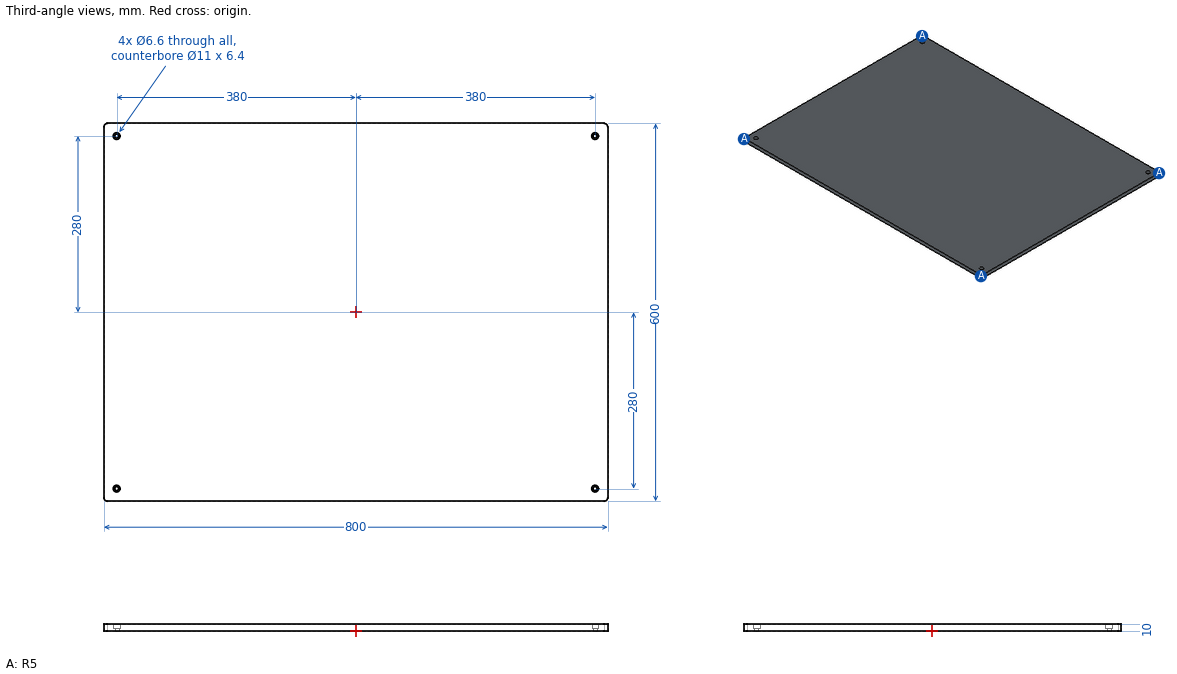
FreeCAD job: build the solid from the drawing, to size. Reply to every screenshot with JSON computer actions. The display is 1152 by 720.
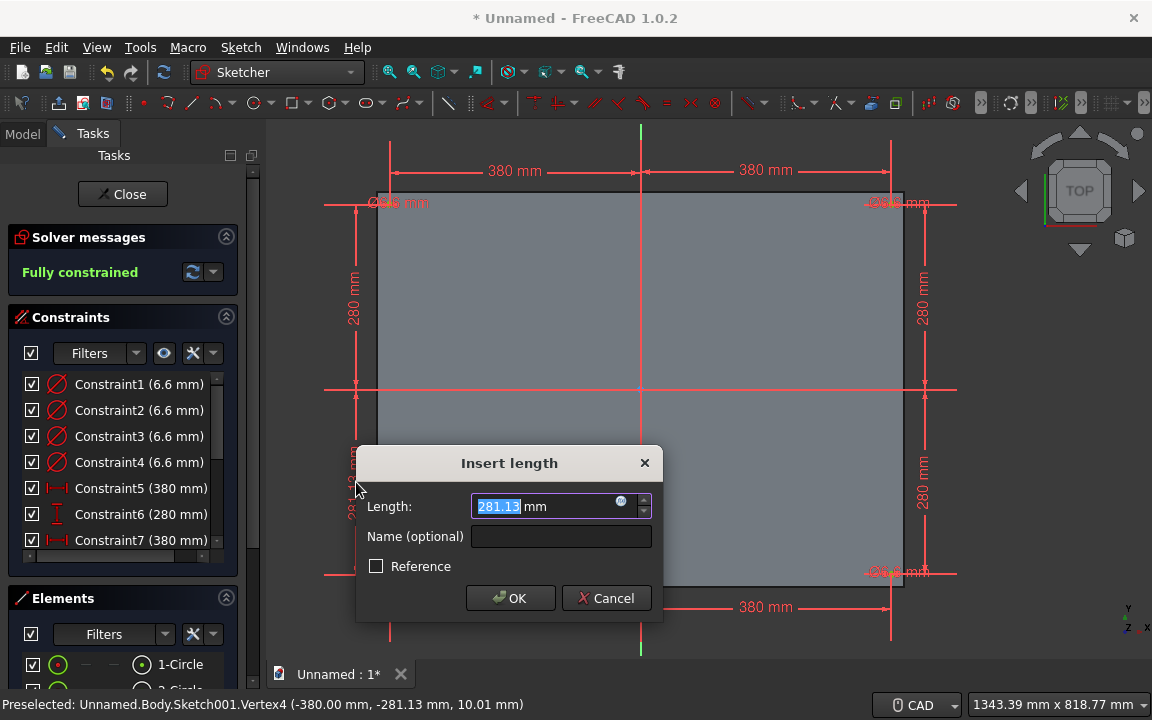
{"action": "type", "text": "280"}
{"action": "key", "text": "Return"}
{"action": "key", "text": "Escape"}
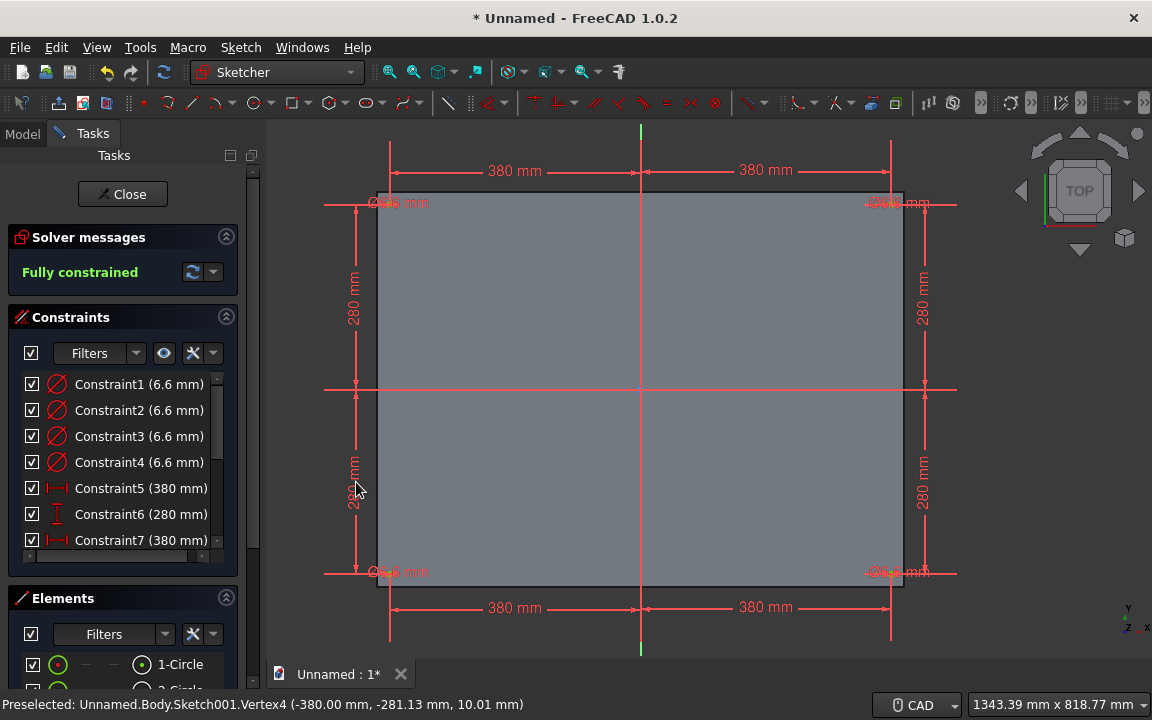
{"action": "left_click", "coordinate": [123, 194]}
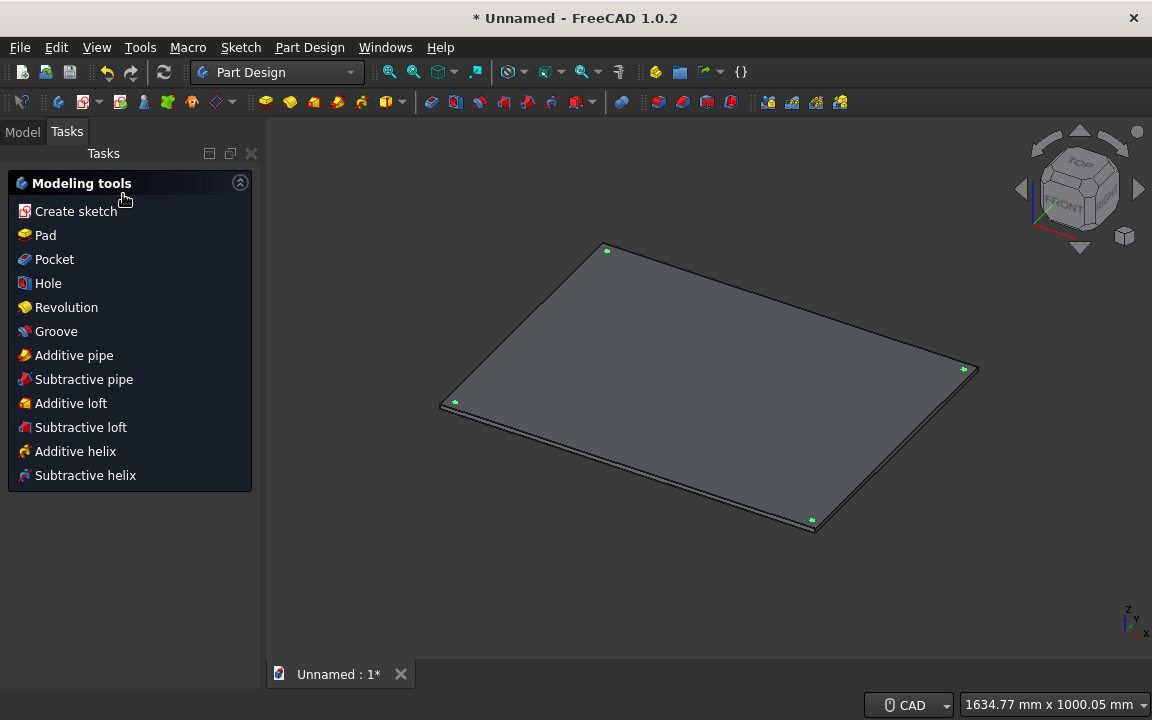
{"action": "left_click", "coordinate": [456, 102]}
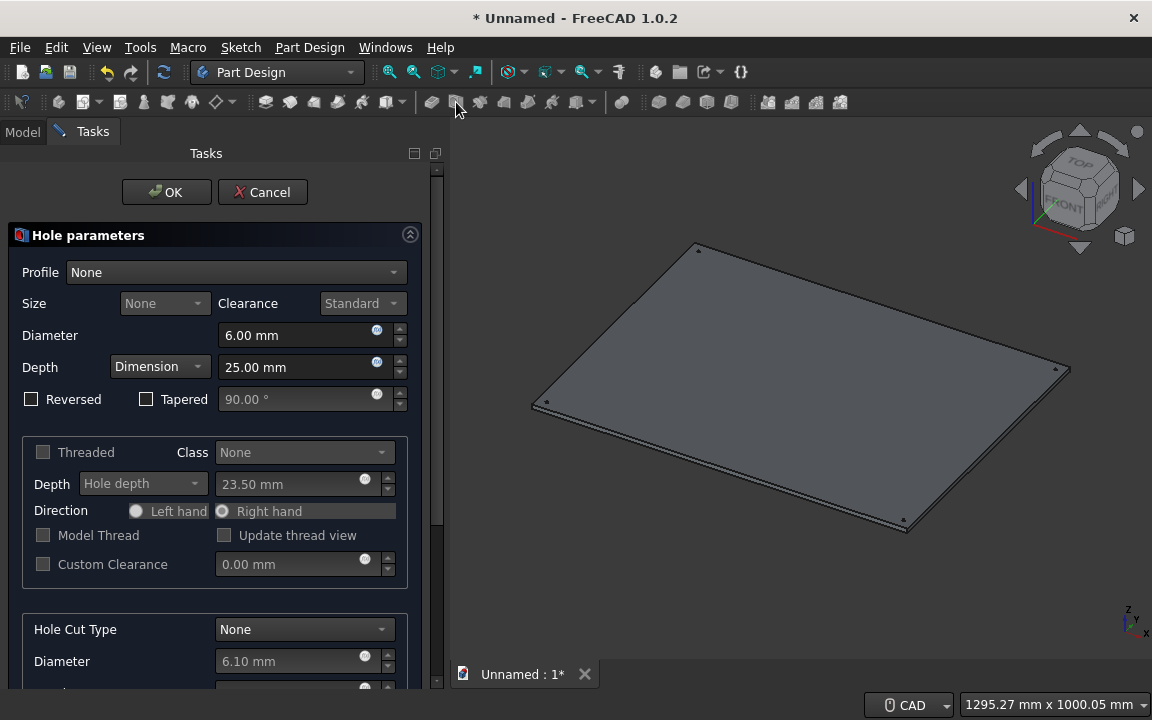
{"action": "triple_click", "coordinate": [305, 335]}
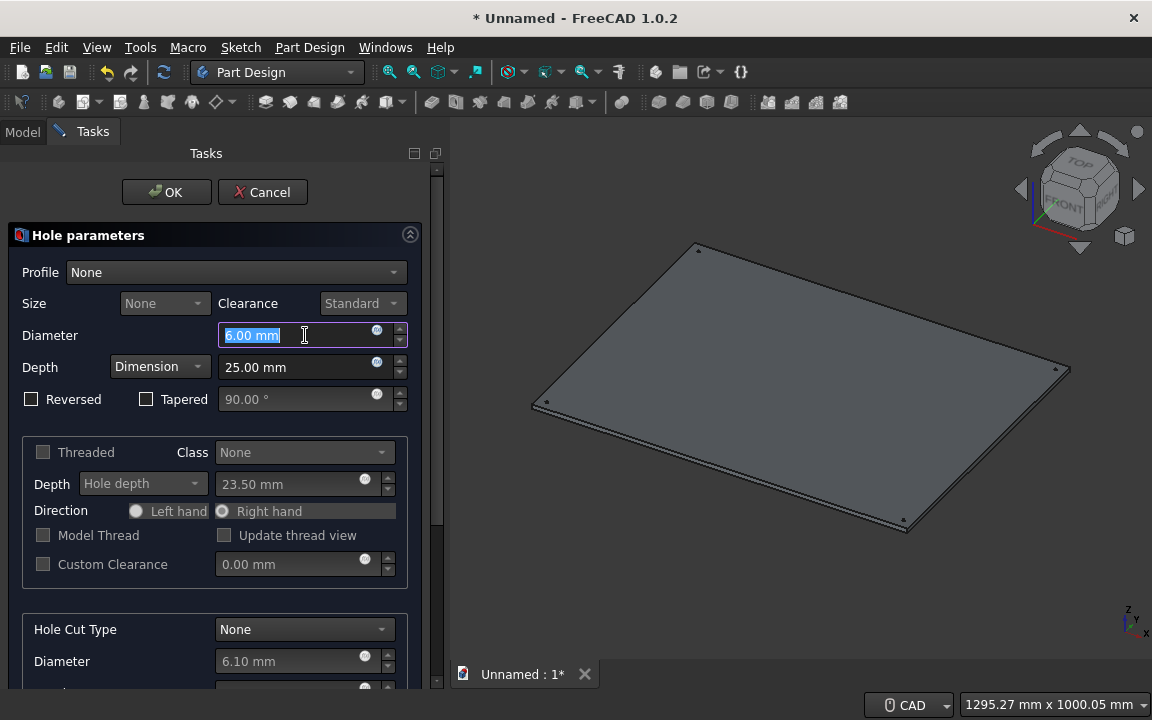
{"action": "type", "text": "6.6"}
{"action": "key", "text": "Tab"}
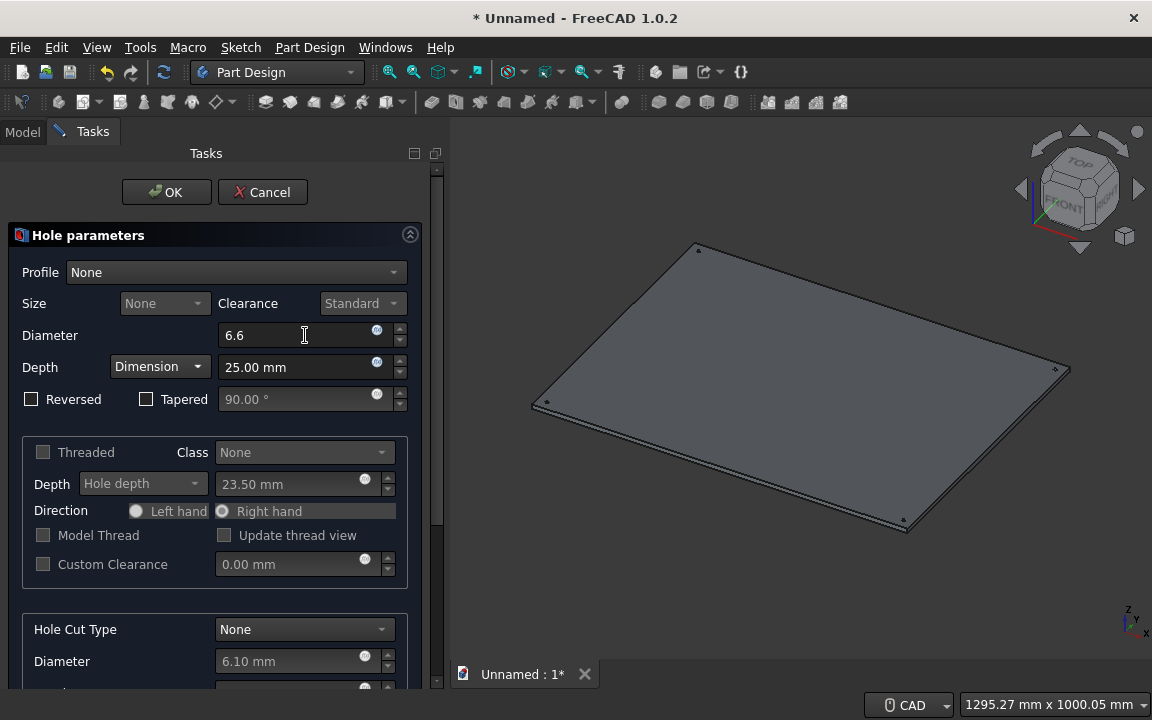
{"action": "left_click", "coordinate": [161, 366]}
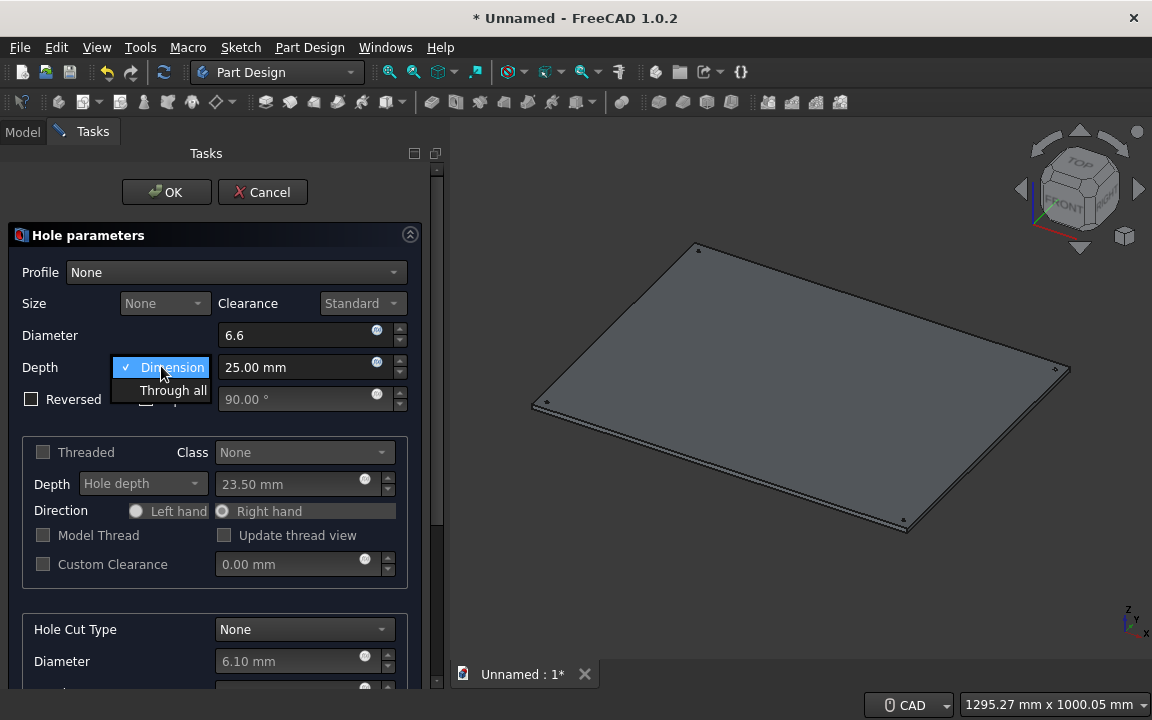
{"action": "left_click", "coordinate": [160, 390]}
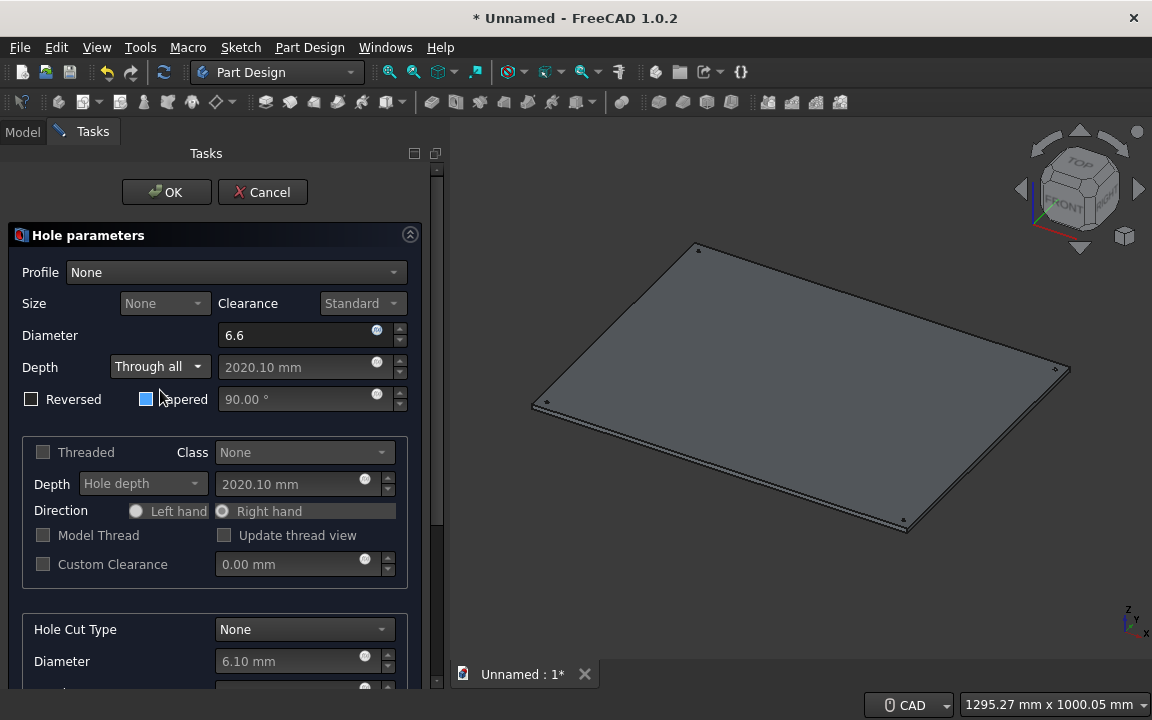
{"action": "left_click", "coordinate": [306, 630]}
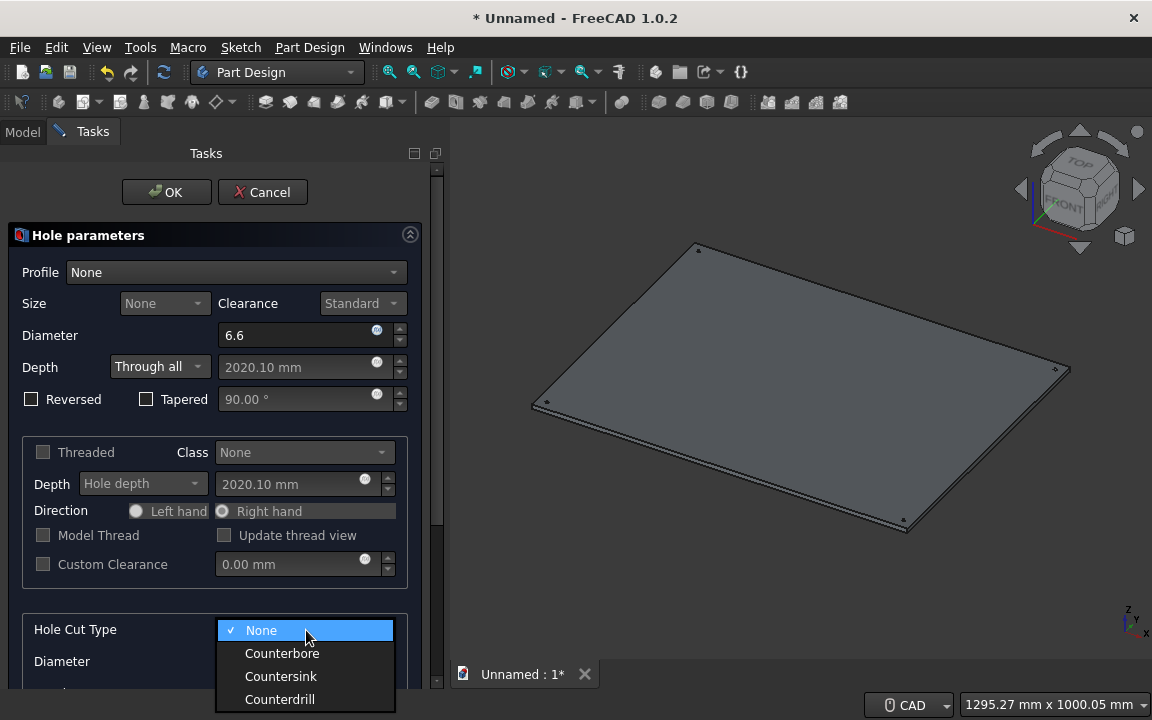
{"action": "left_click", "coordinate": [304, 654]}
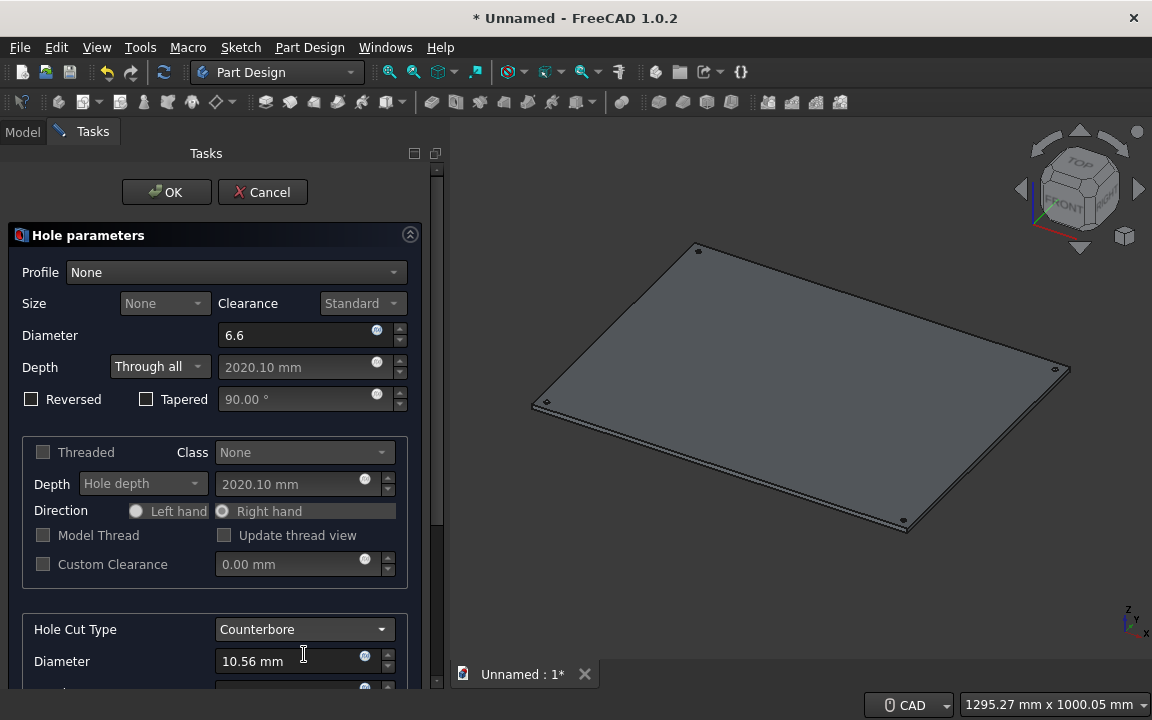
{"action": "triple_click", "coordinate": [298, 661]}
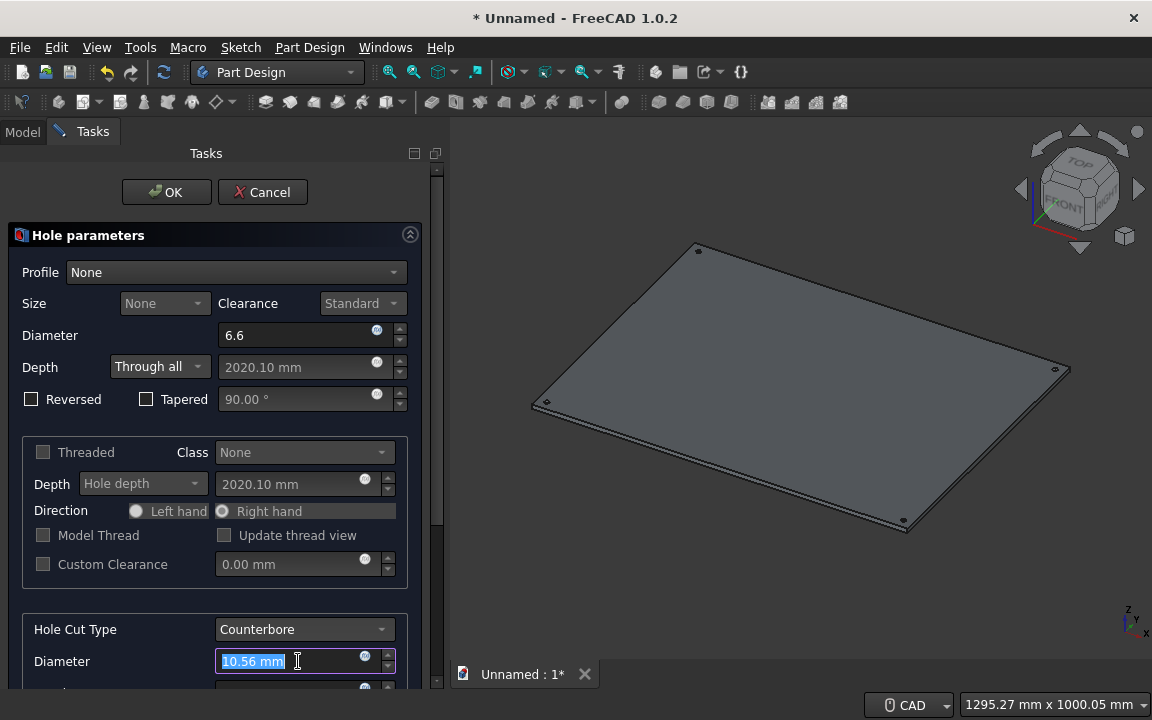
{"action": "type", "text": "11"}
{"action": "key", "text": "Tab"}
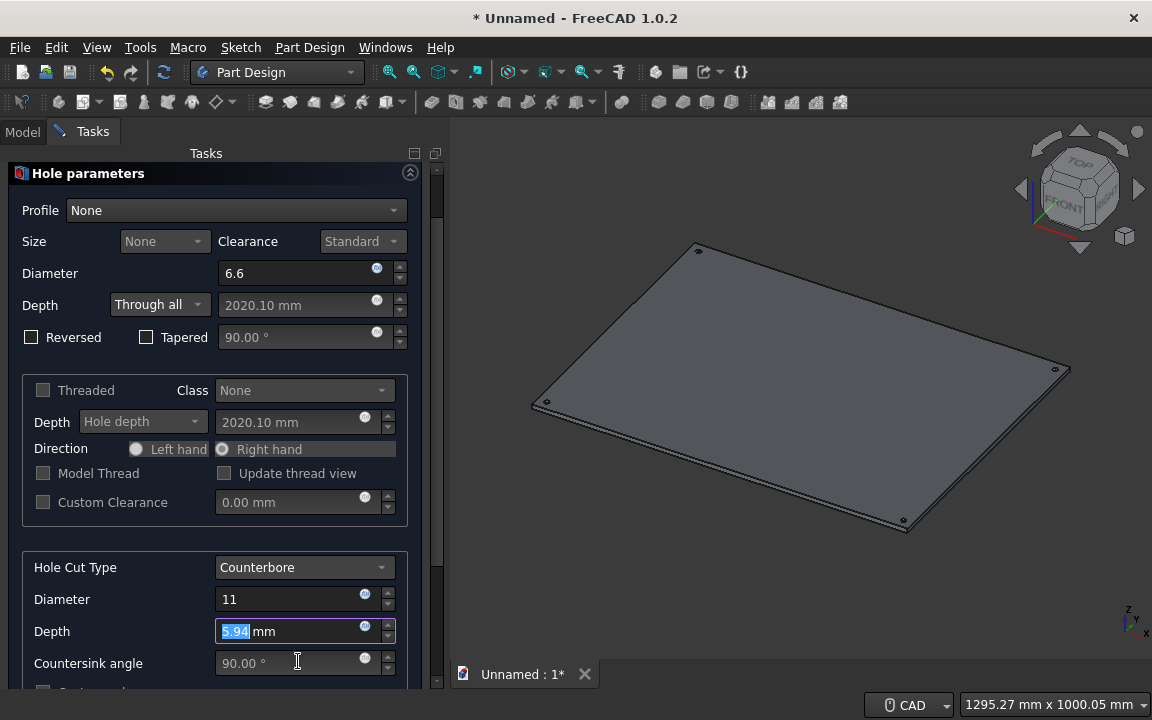
{"action": "type", "text": "6.4"}
{"action": "key", "text": "Tab"}